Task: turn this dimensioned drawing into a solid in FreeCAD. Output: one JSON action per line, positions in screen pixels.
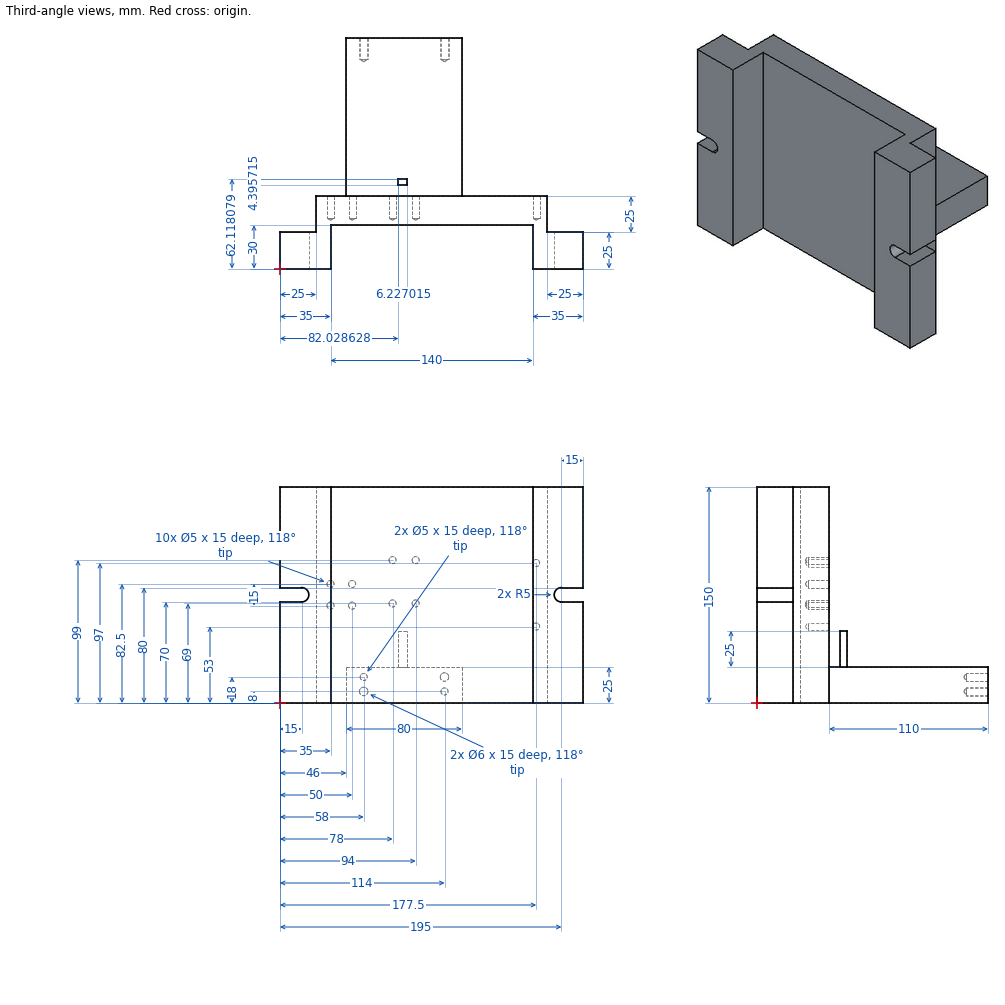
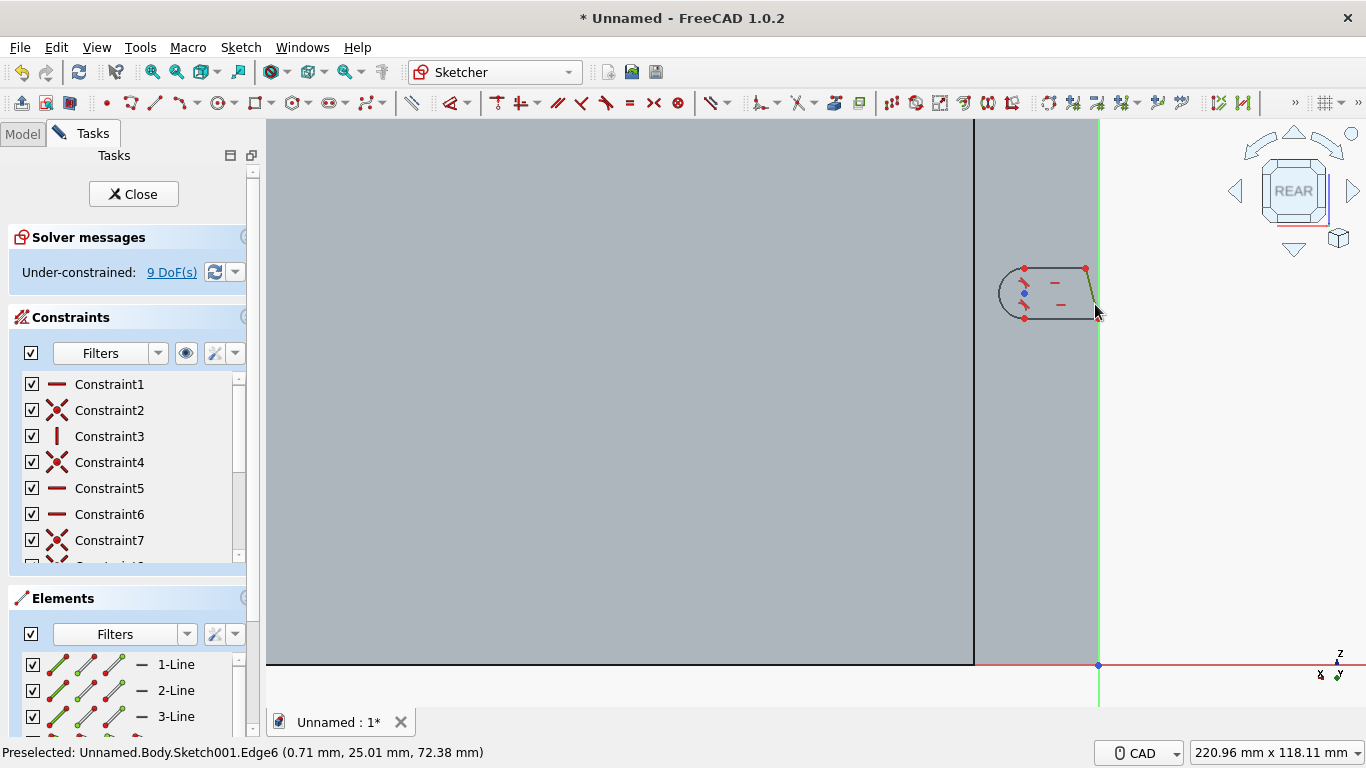
{"action": "left_click", "coordinate": [540, 104]}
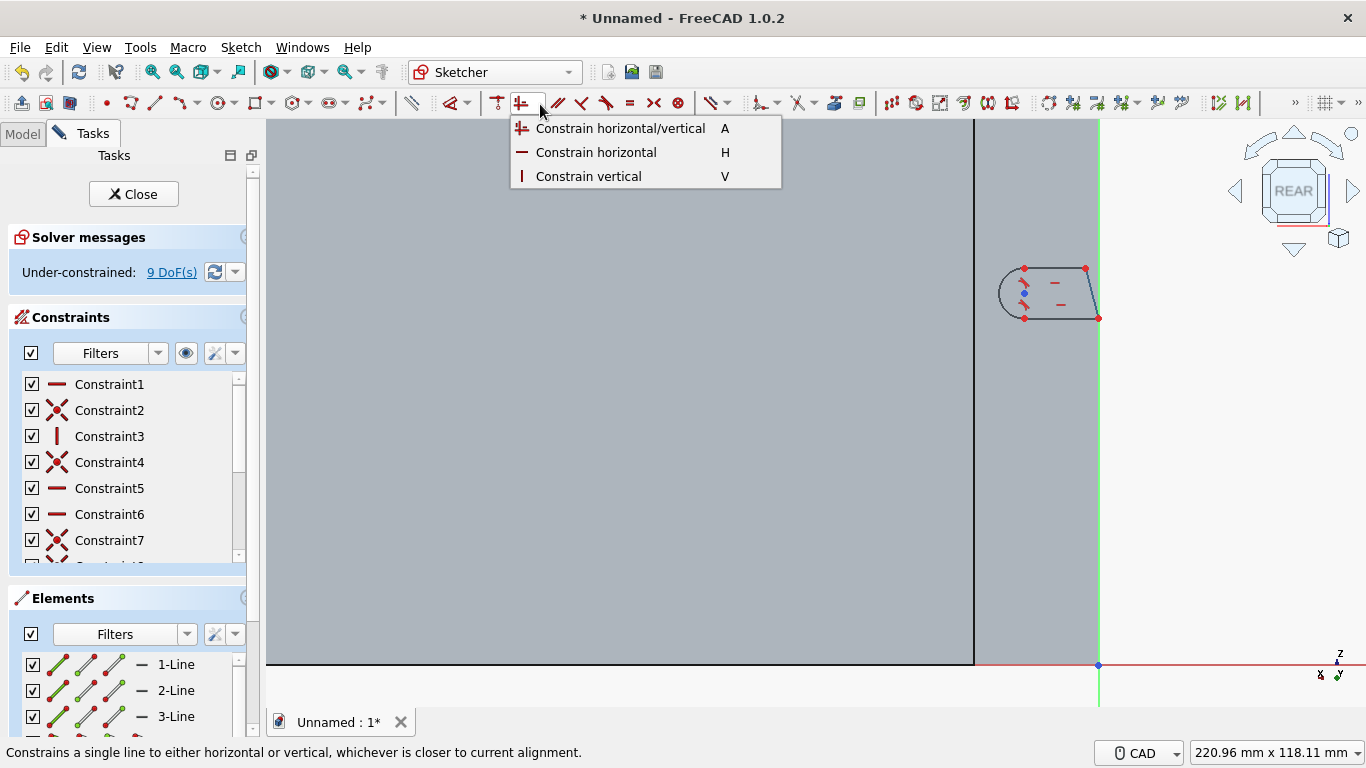
{"action": "left_click", "coordinate": [646, 176]}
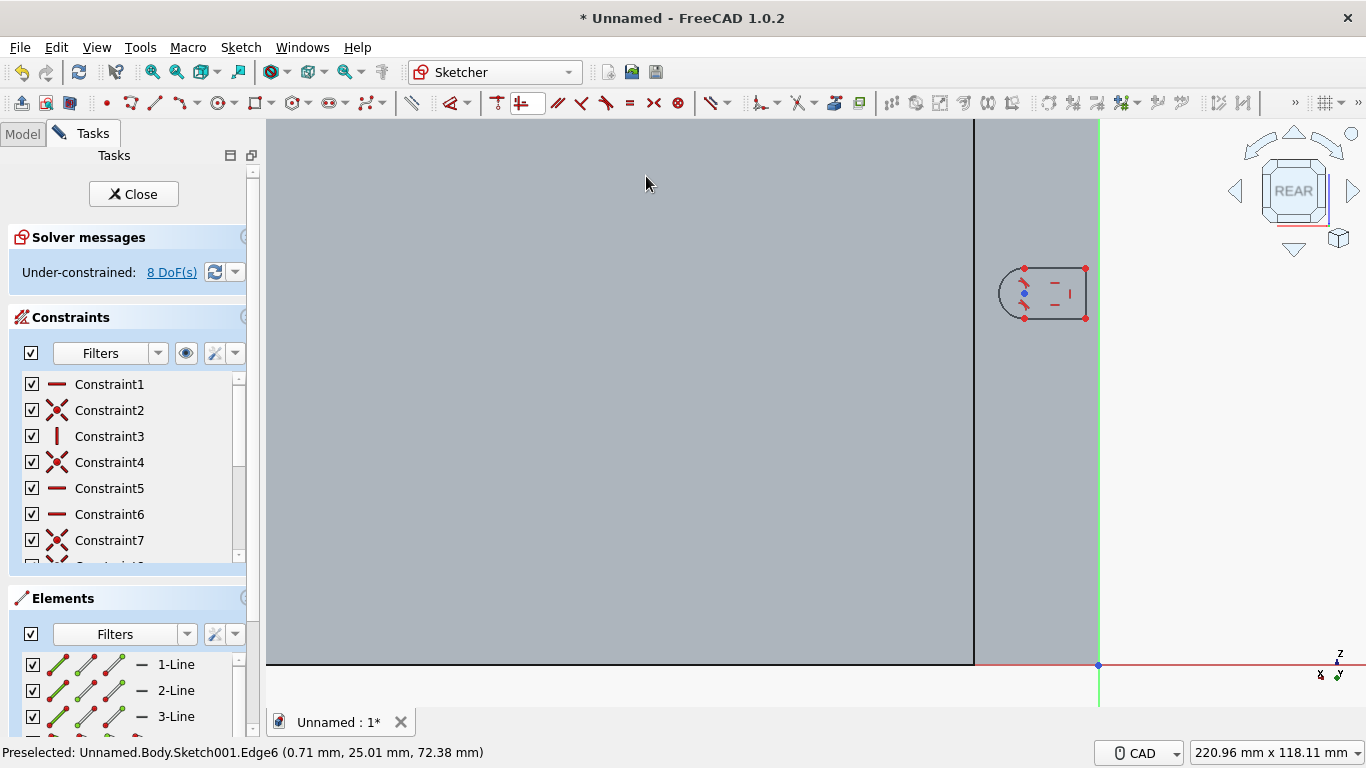
{"action": "scroll", "coordinate": [1096, 305], "scroll_direction": "down", "scroll_amount": 2}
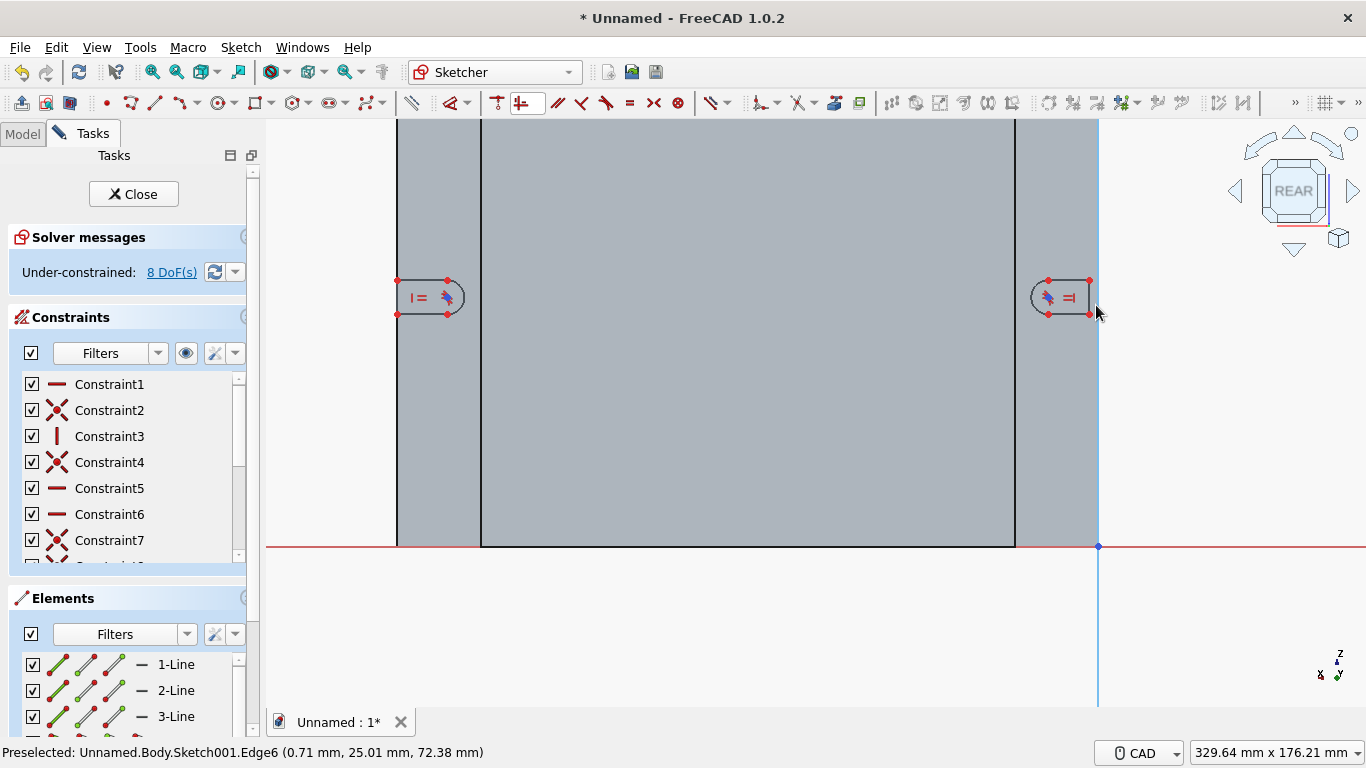
{"action": "left_click", "coordinate": [461, 307]}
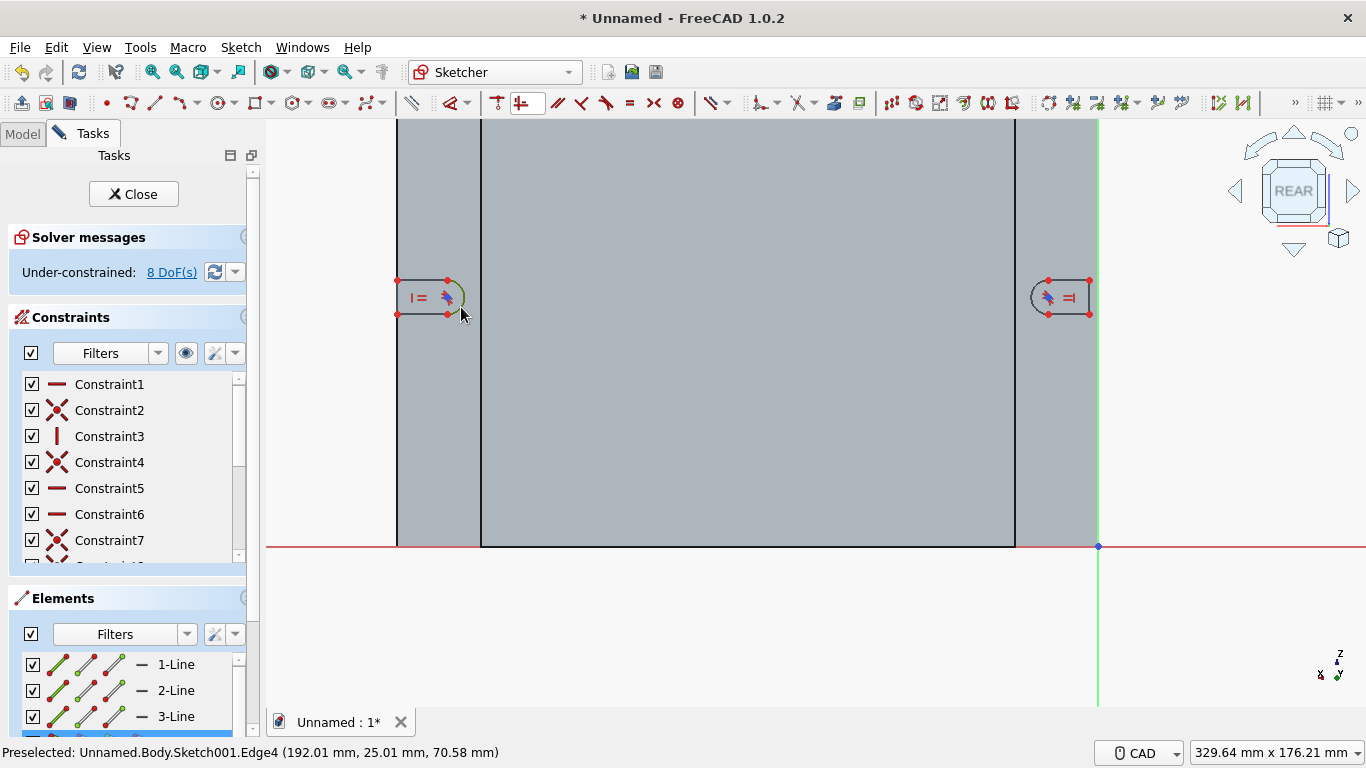
{"action": "left_click", "coordinate": [1035, 287]}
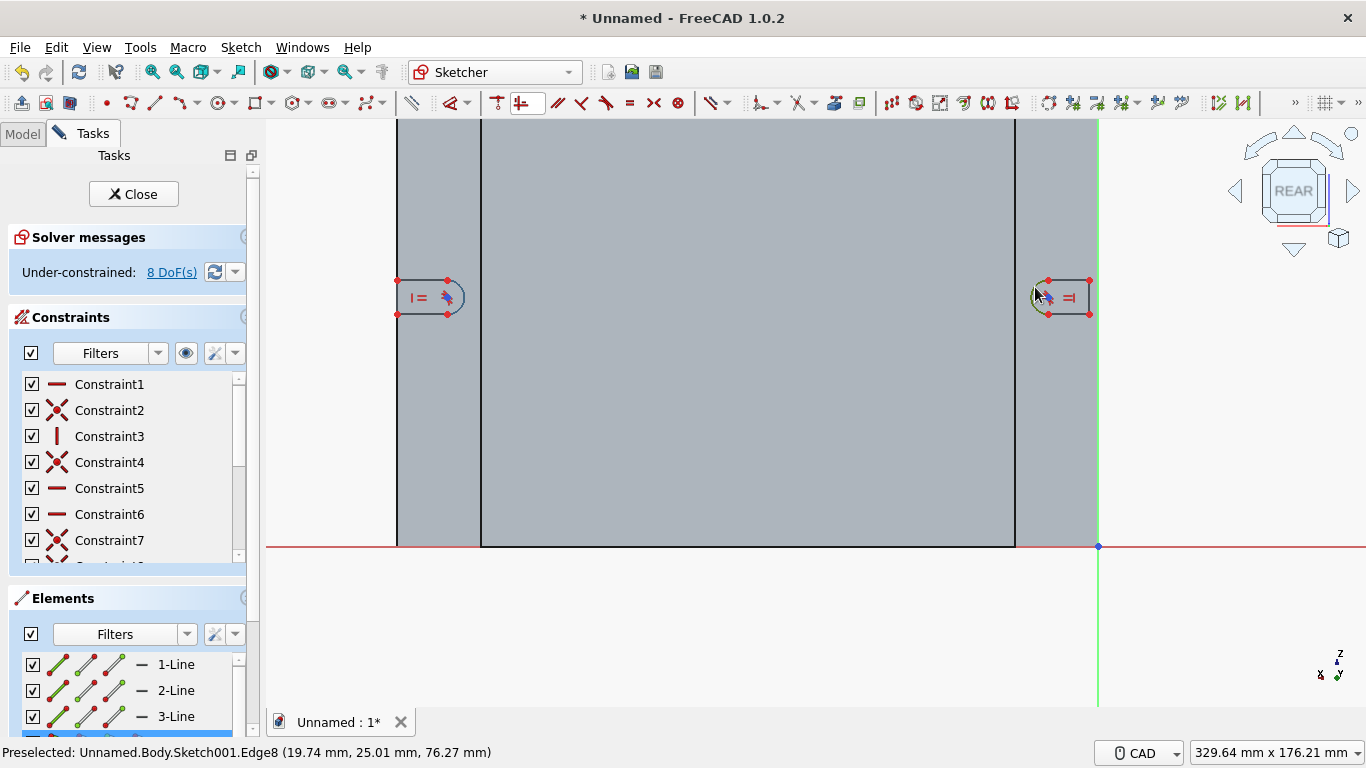
{"action": "key", "text": "e"}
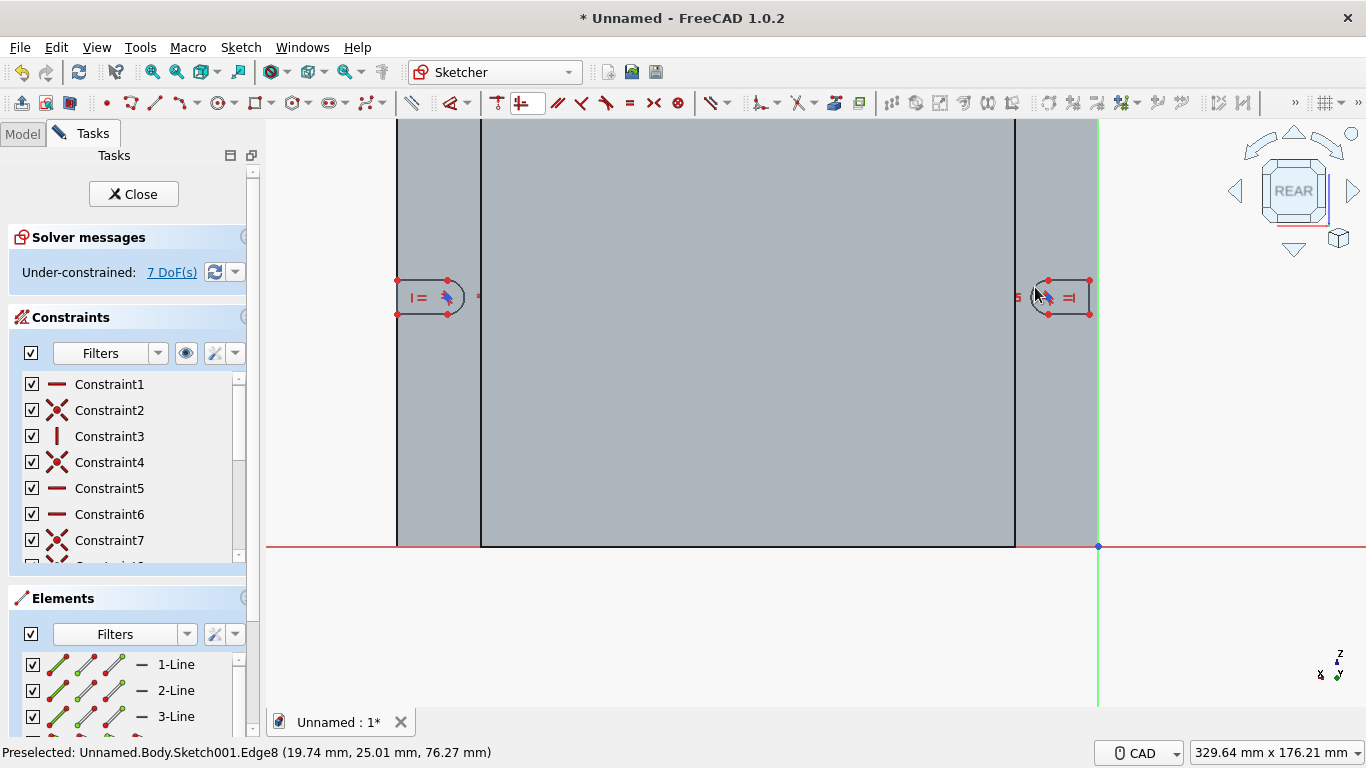
{"action": "key", "text": "d"}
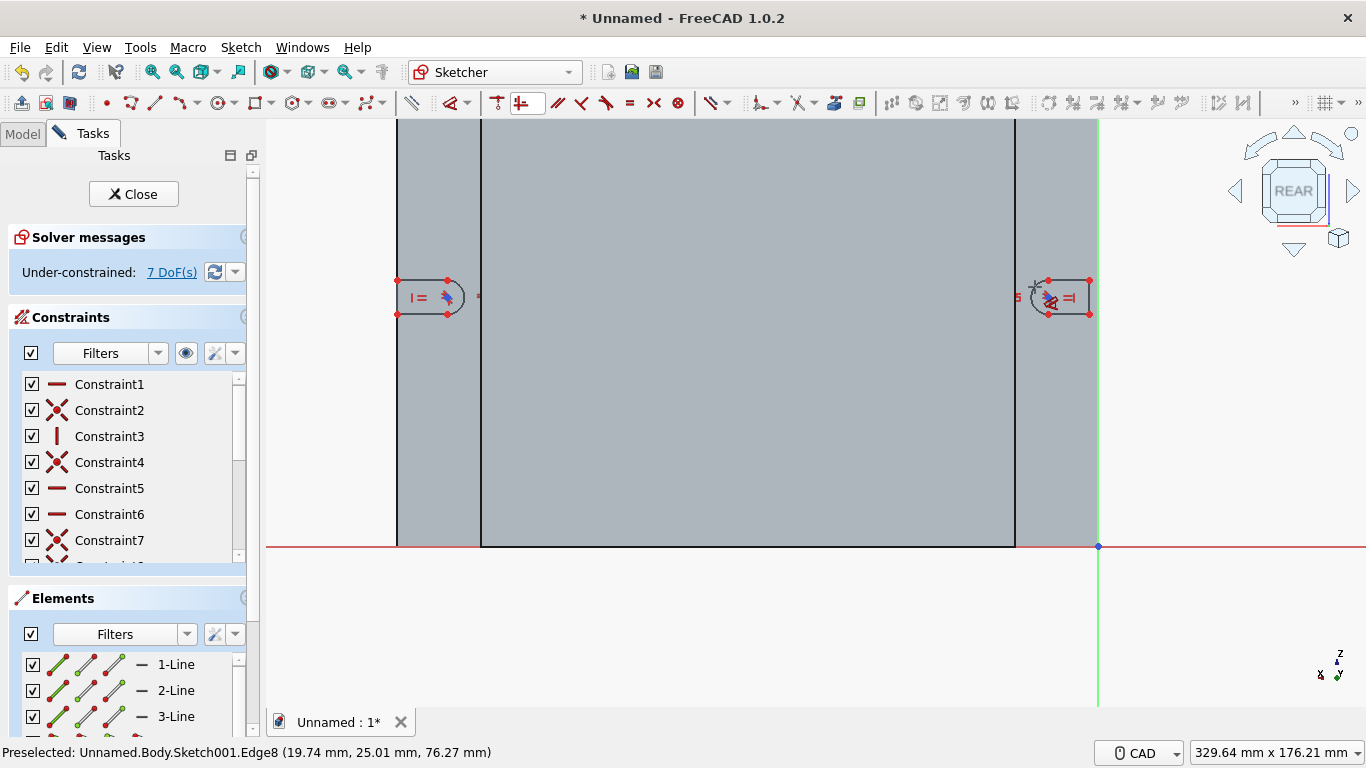
{"action": "scroll", "coordinate": [461, 307], "scroll_direction": "up", "scroll_amount": 5}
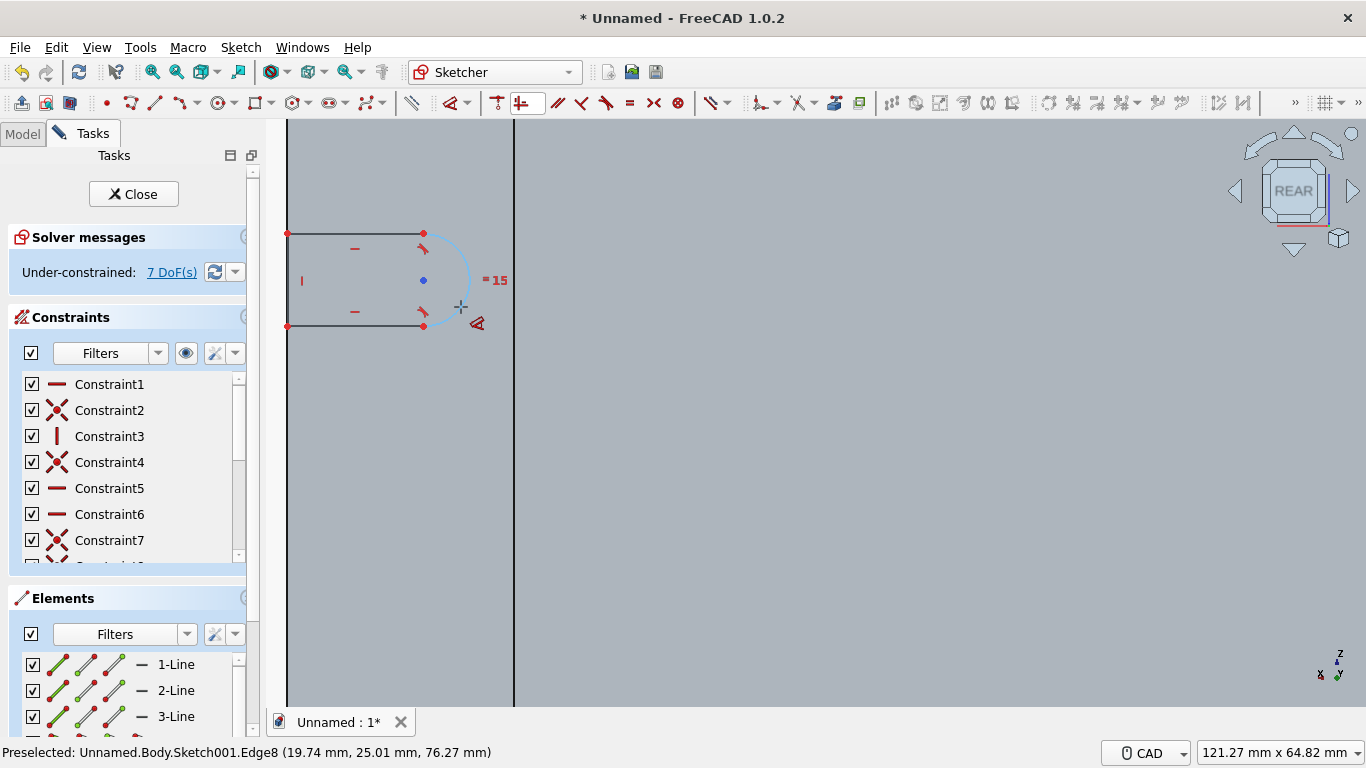
{"action": "left_click", "coordinate": [461, 307]}
{"action": "left_click", "coordinate": [487, 326]}